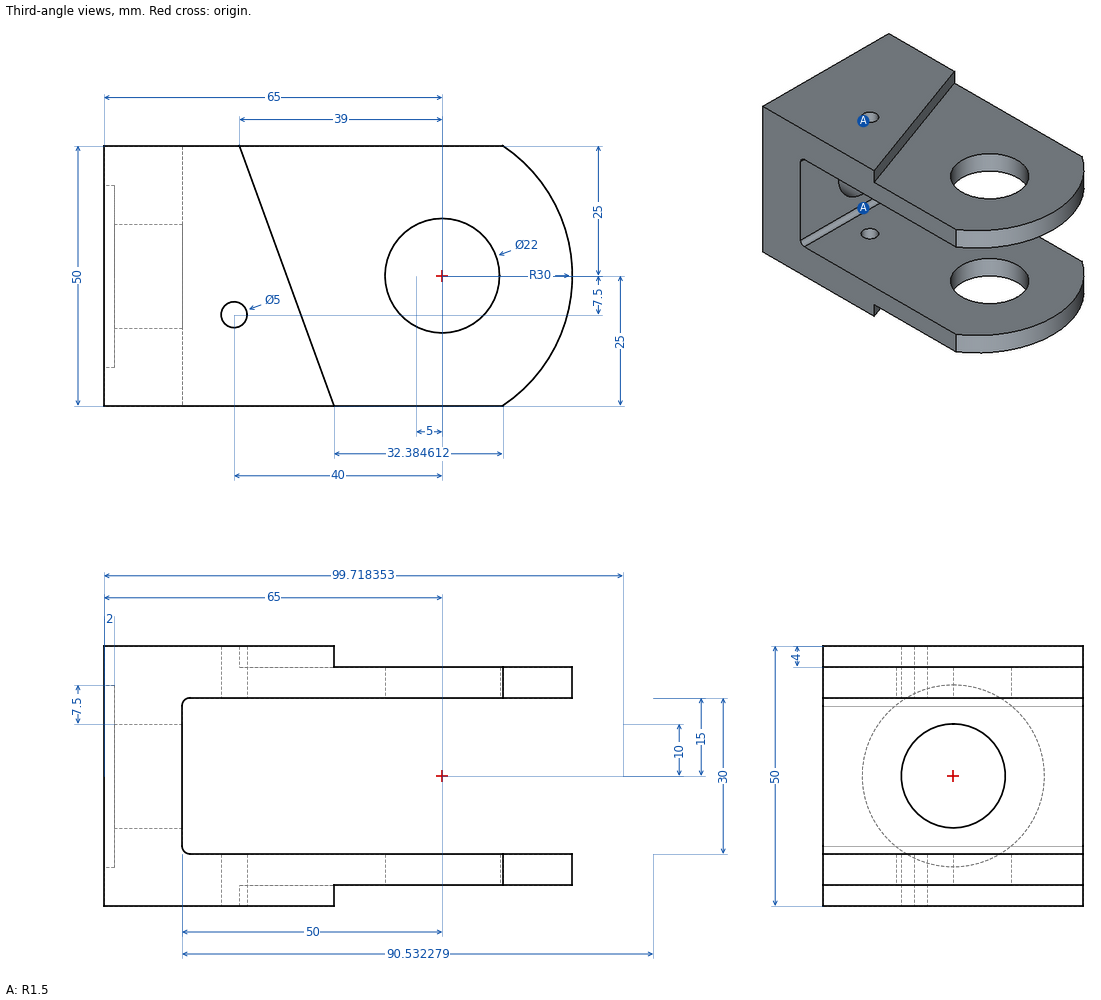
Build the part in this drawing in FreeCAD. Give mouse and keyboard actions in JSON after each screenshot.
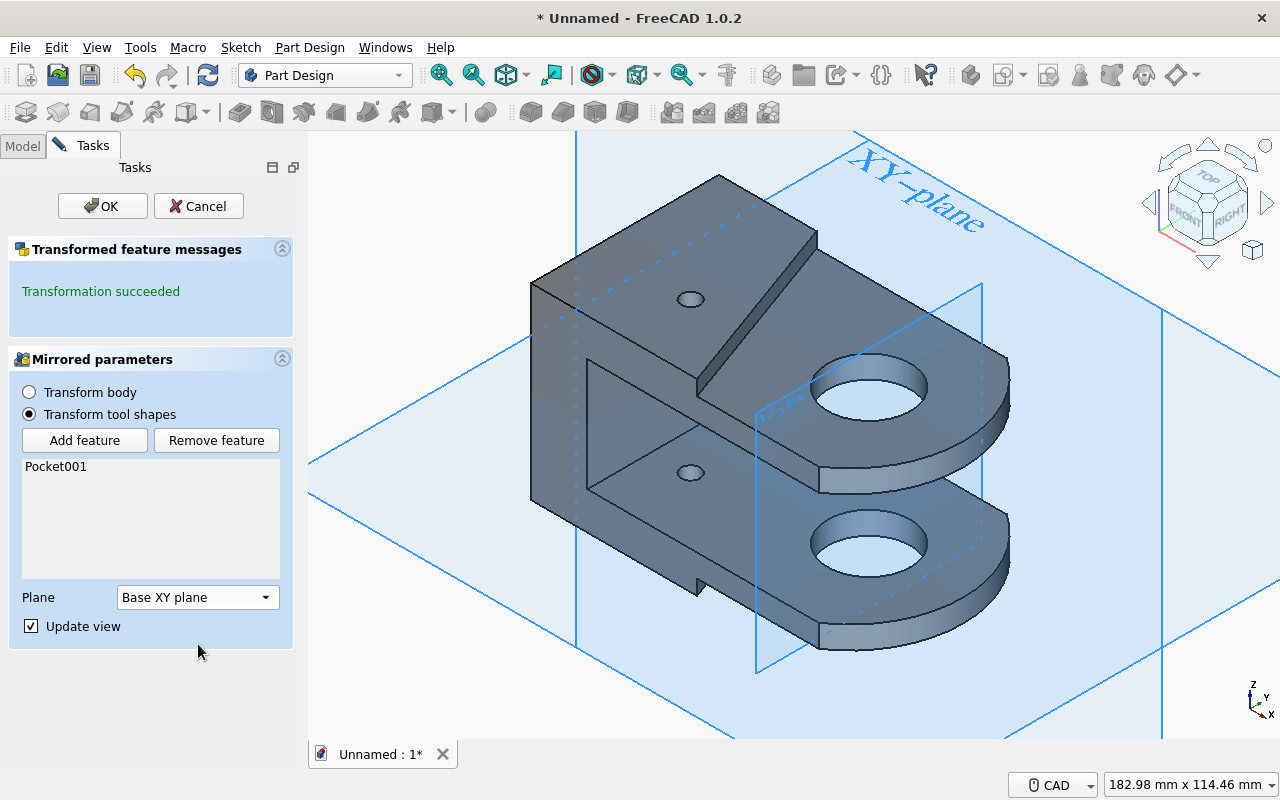
{"action": "left_click", "coordinate": [103, 206]}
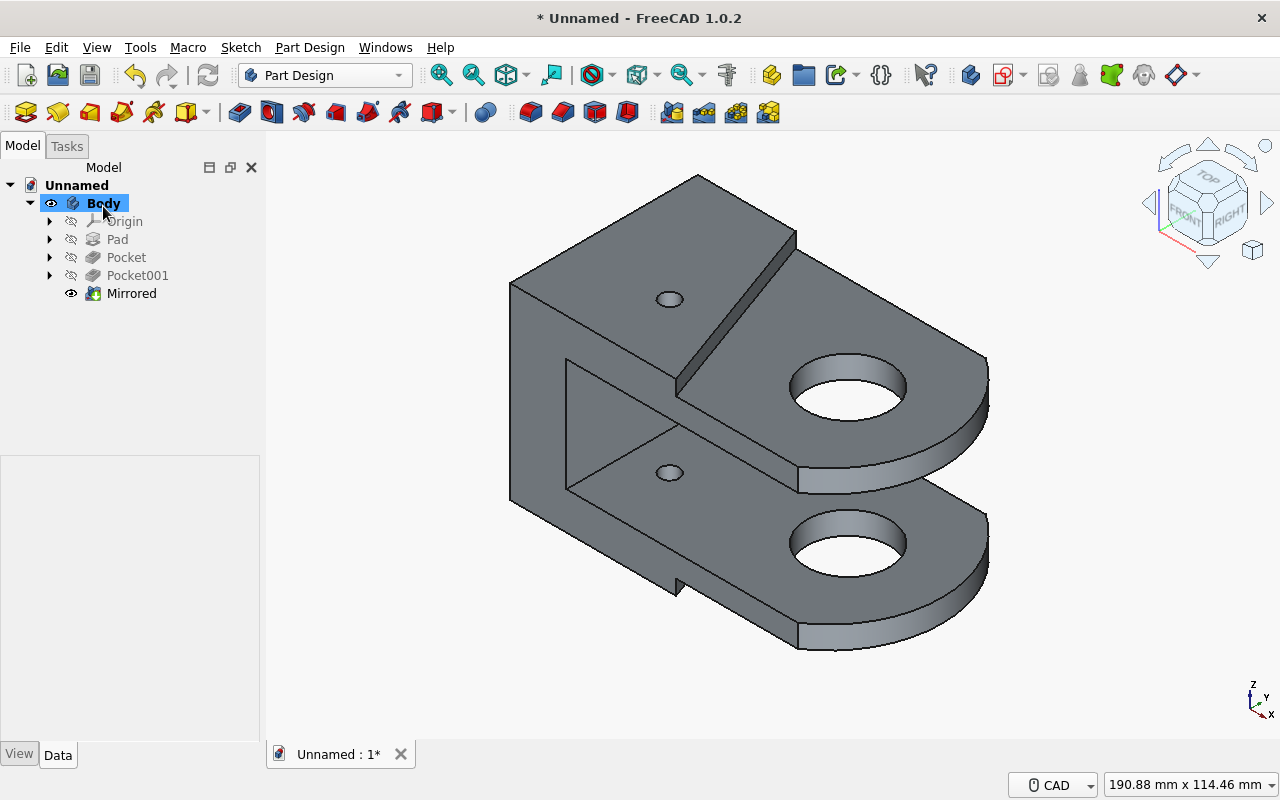
{"action": "key", "text": "2"}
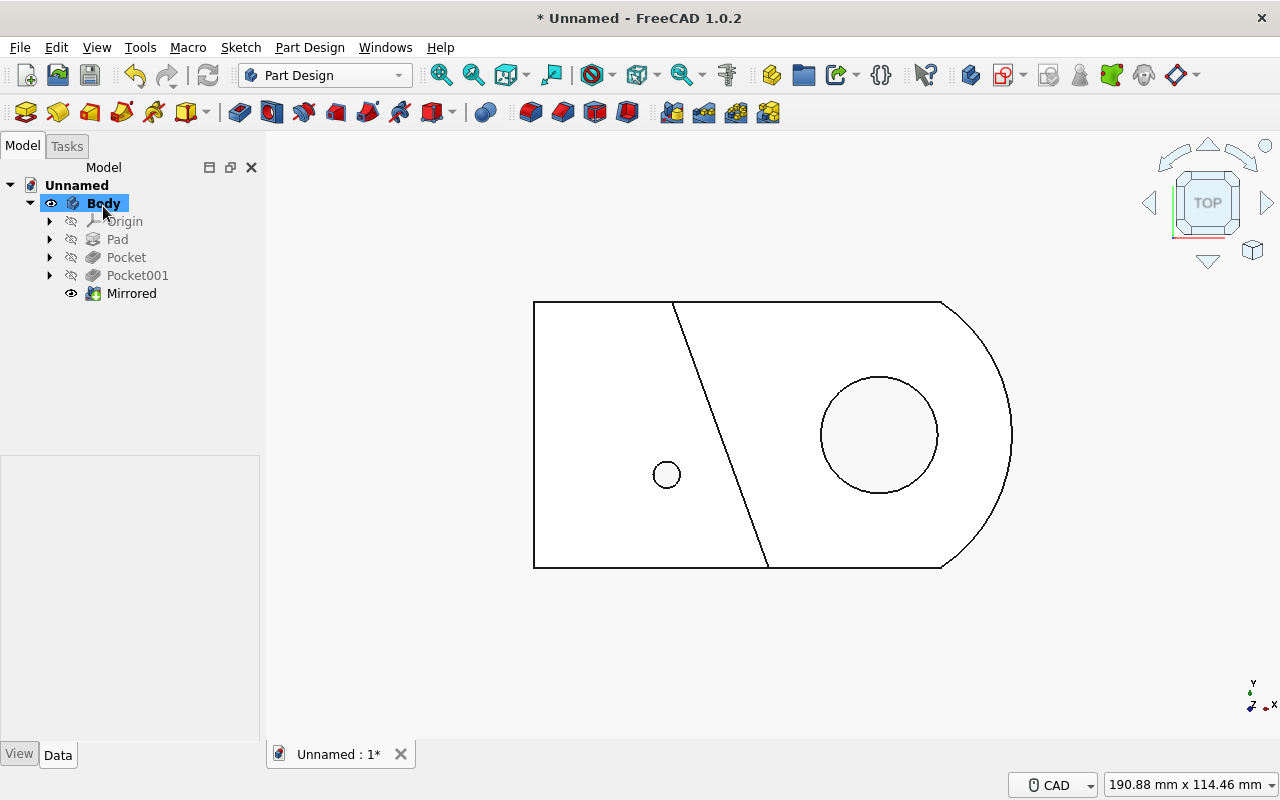
{"action": "key", "text": "0"}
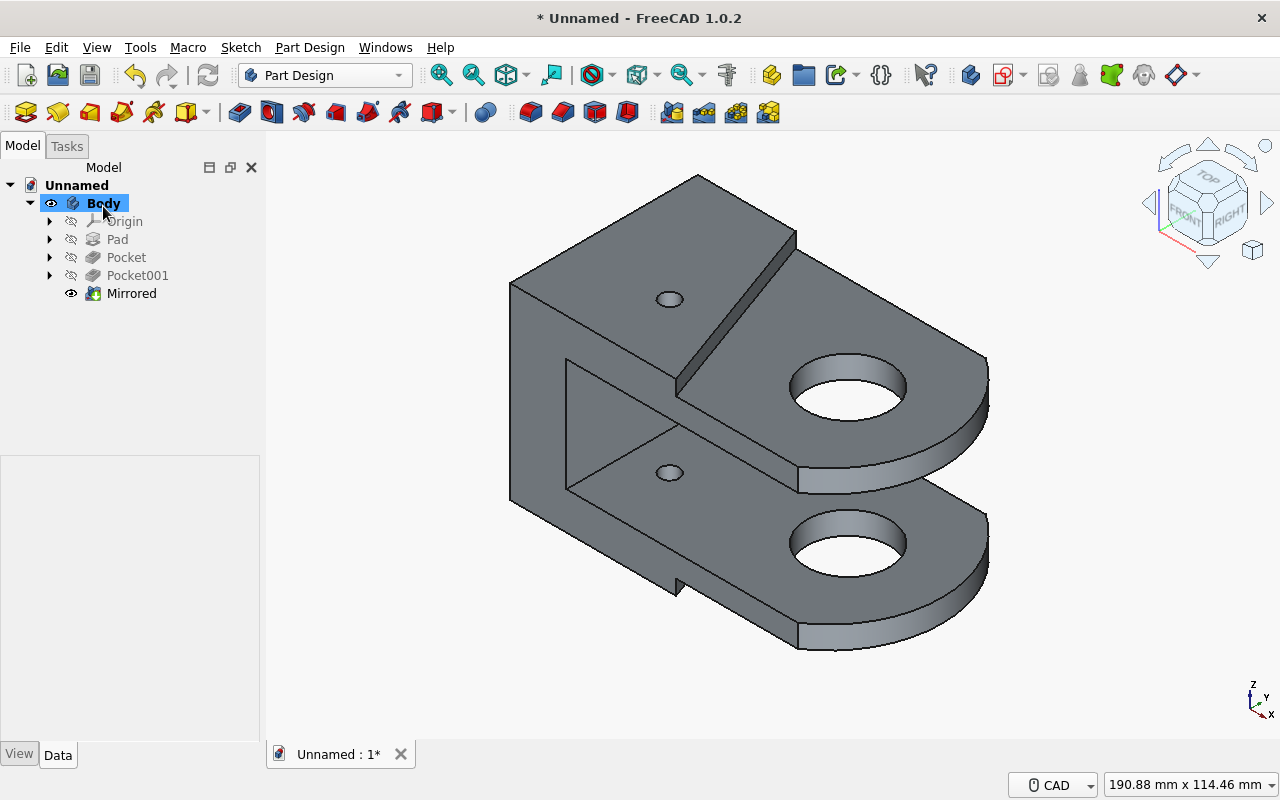
{"action": "key", "text": "1"}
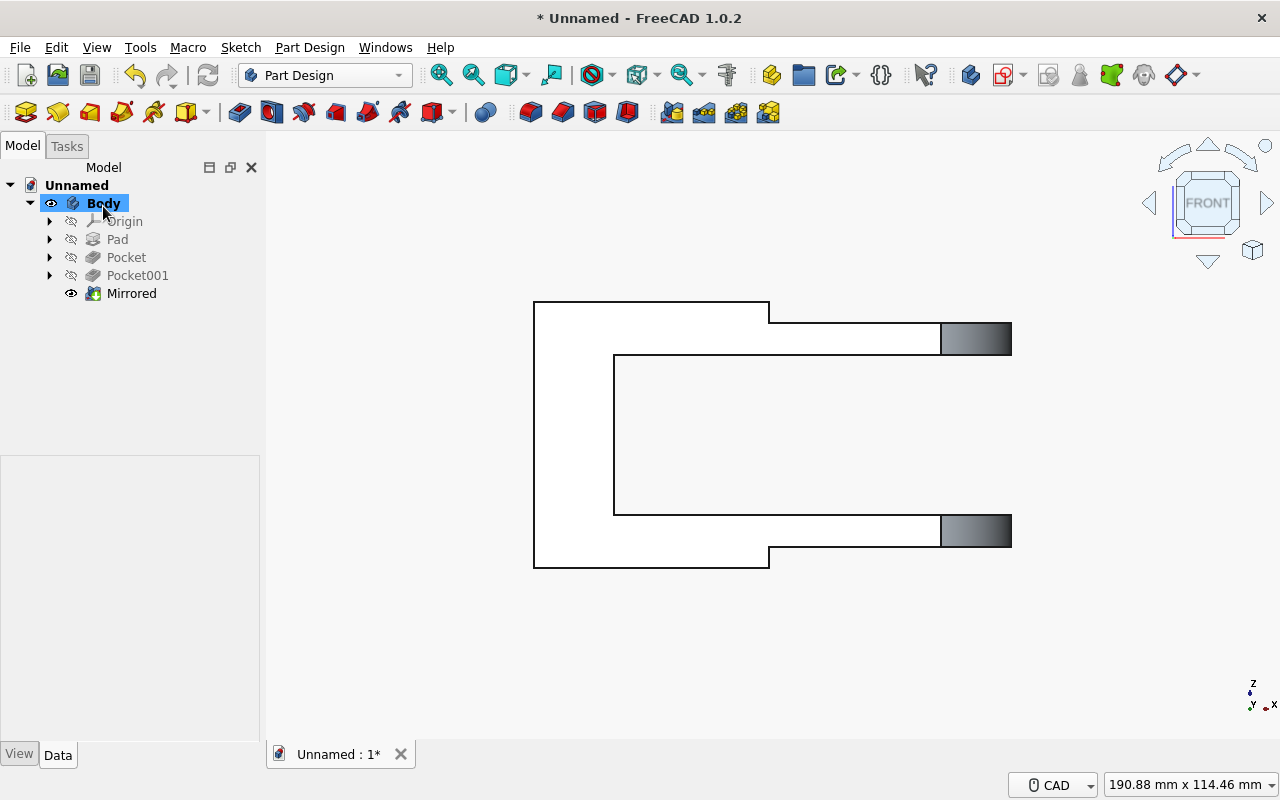
{"action": "key", "text": "3"}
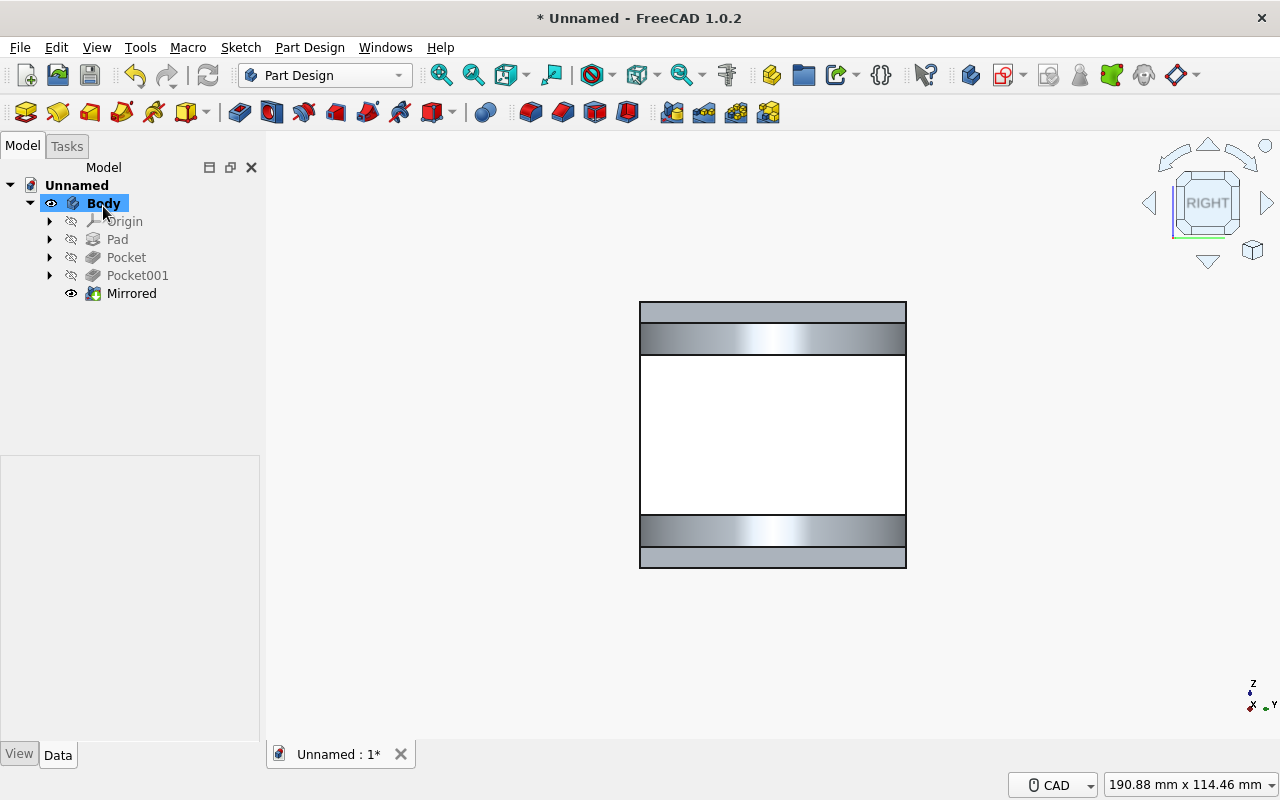
{"action": "left_click", "coordinate": [442, 76]}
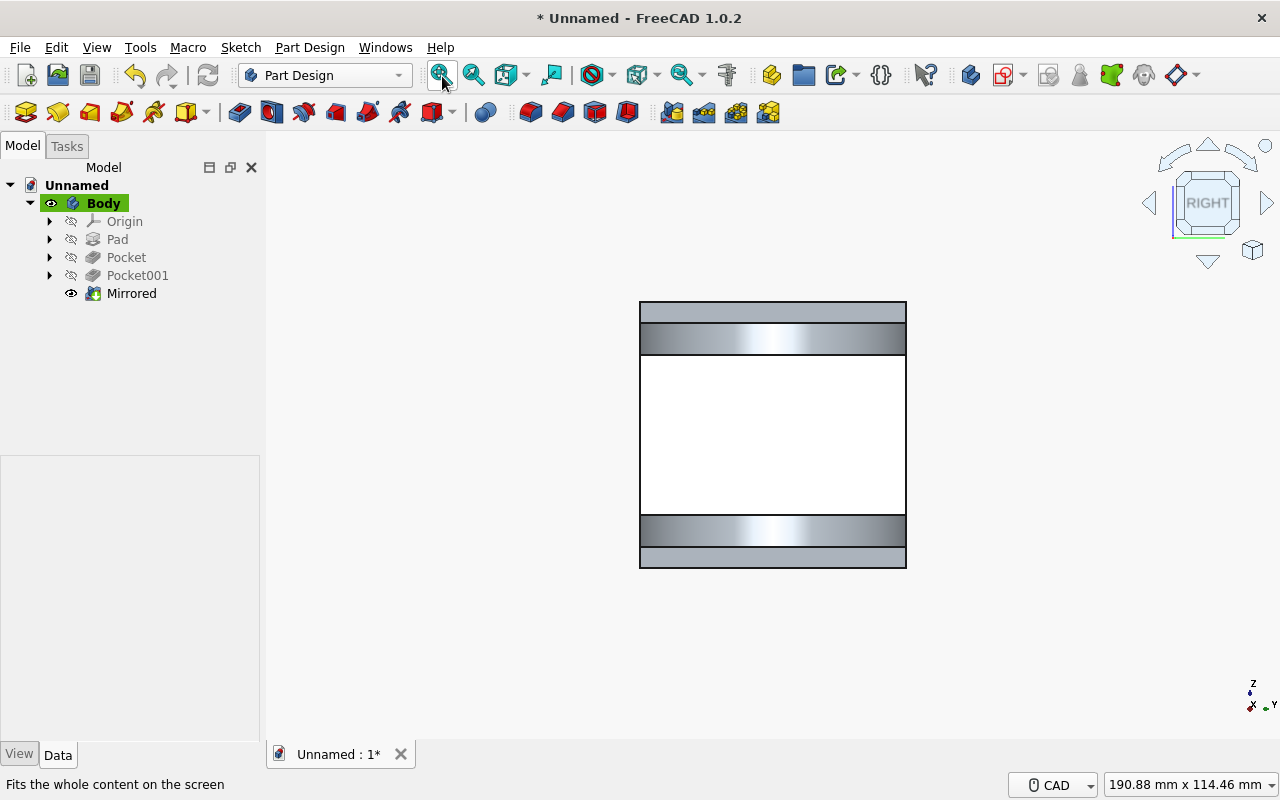
{"action": "key", "text": "5"}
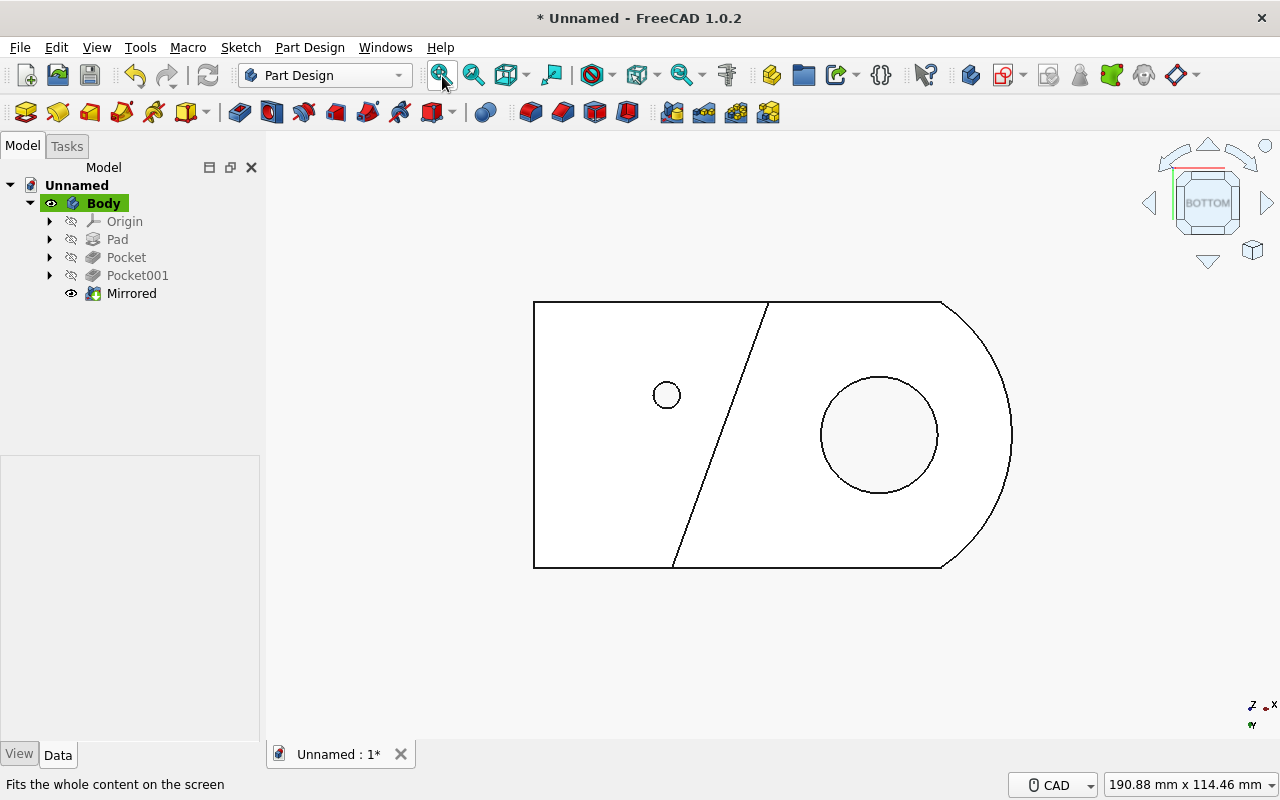
{"action": "key", "text": "4"}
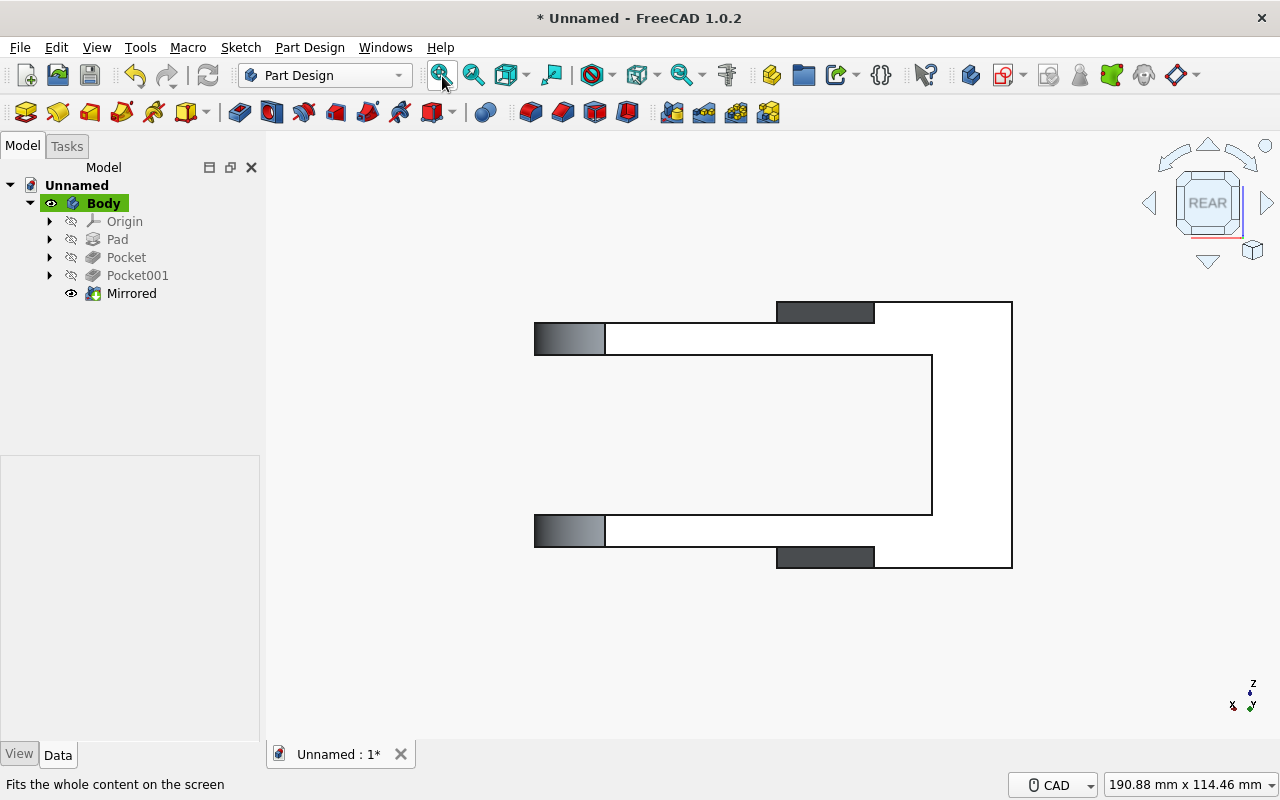
{"action": "key", "text": "6"}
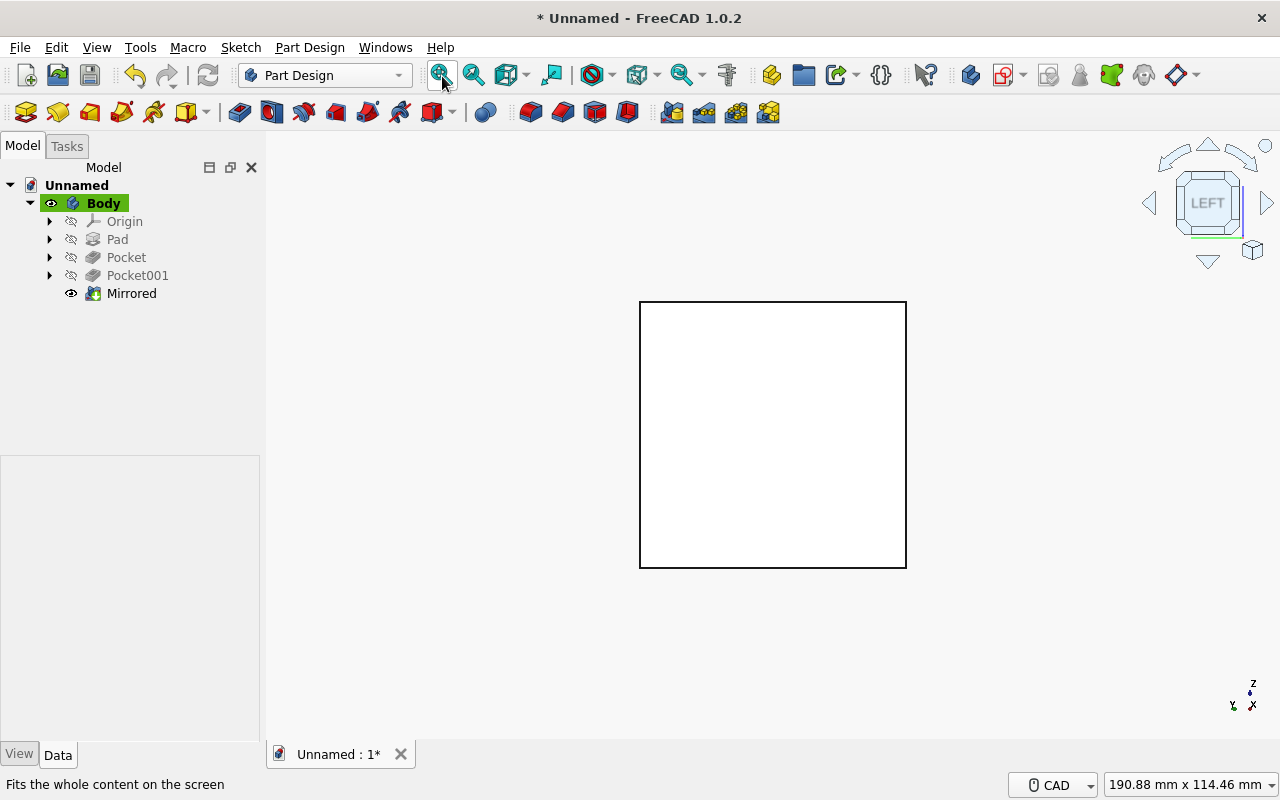
{"action": "left_click", "coordinate": [442, 76]}